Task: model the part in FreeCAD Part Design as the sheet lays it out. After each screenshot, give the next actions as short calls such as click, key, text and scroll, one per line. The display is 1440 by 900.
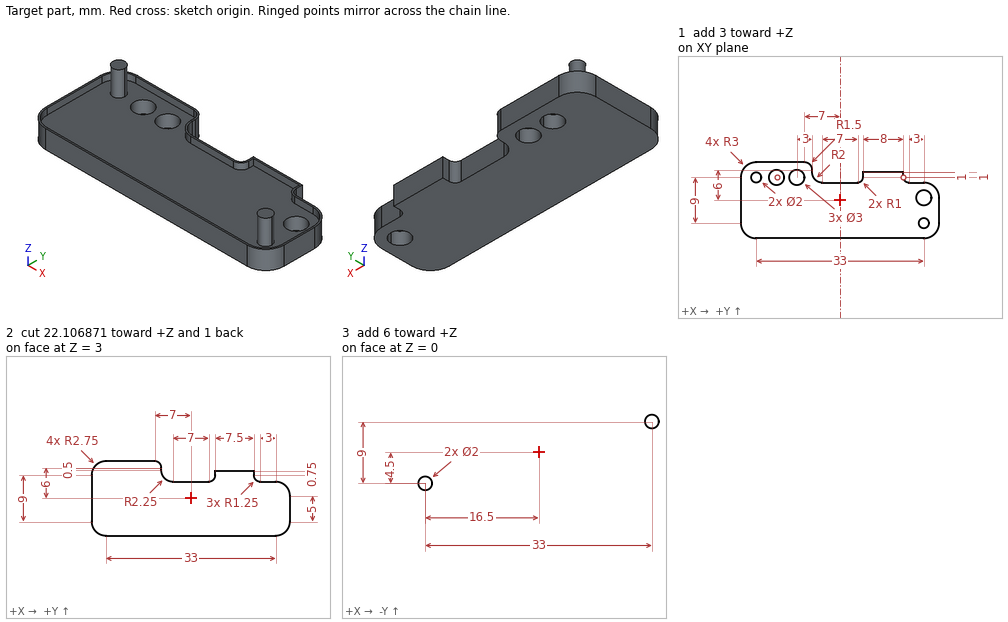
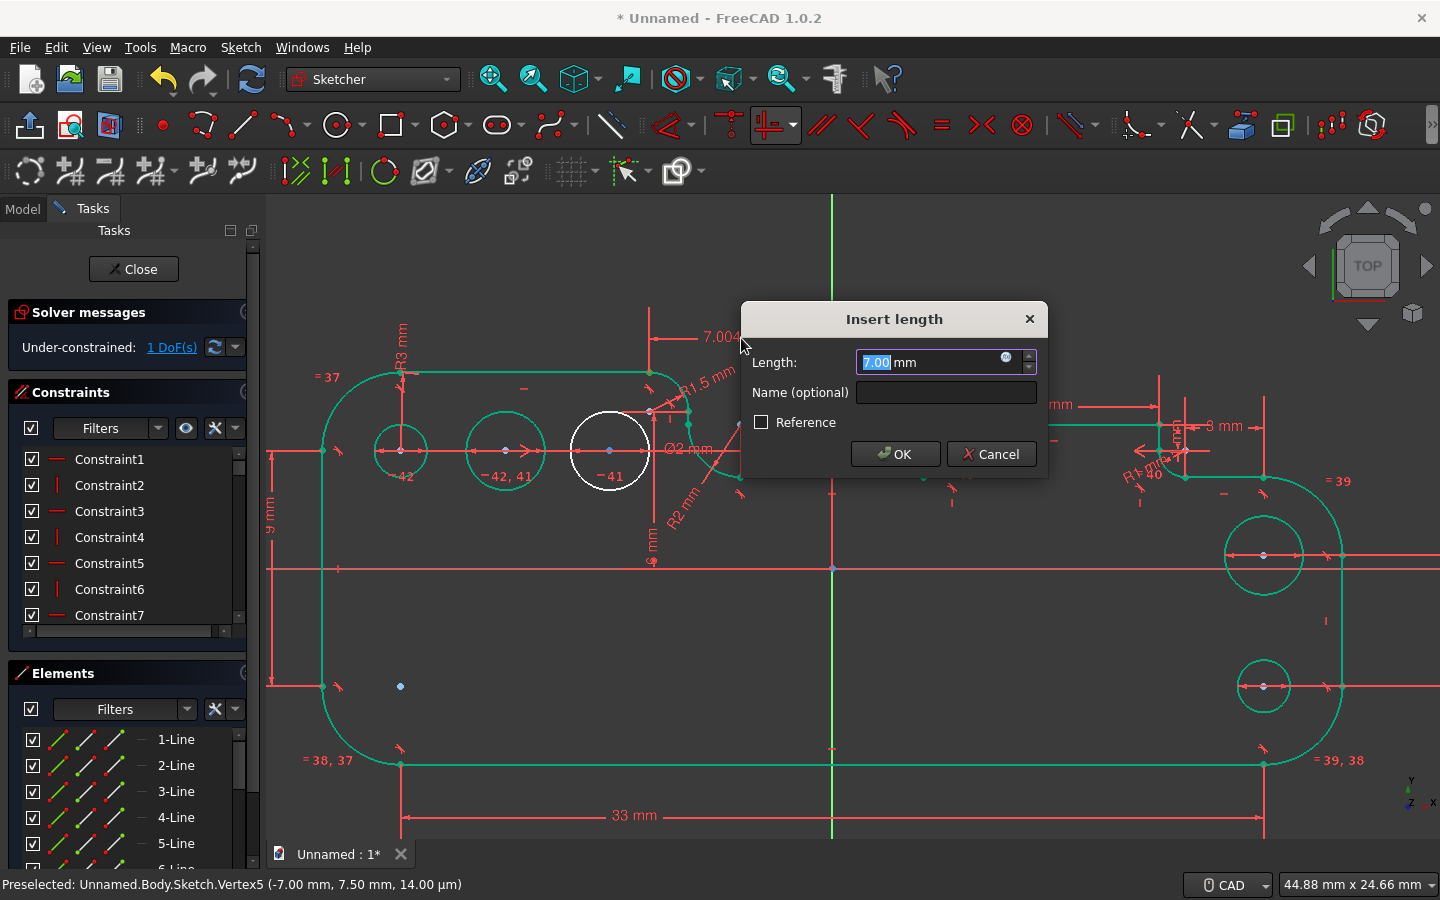
text(7)
key(Return)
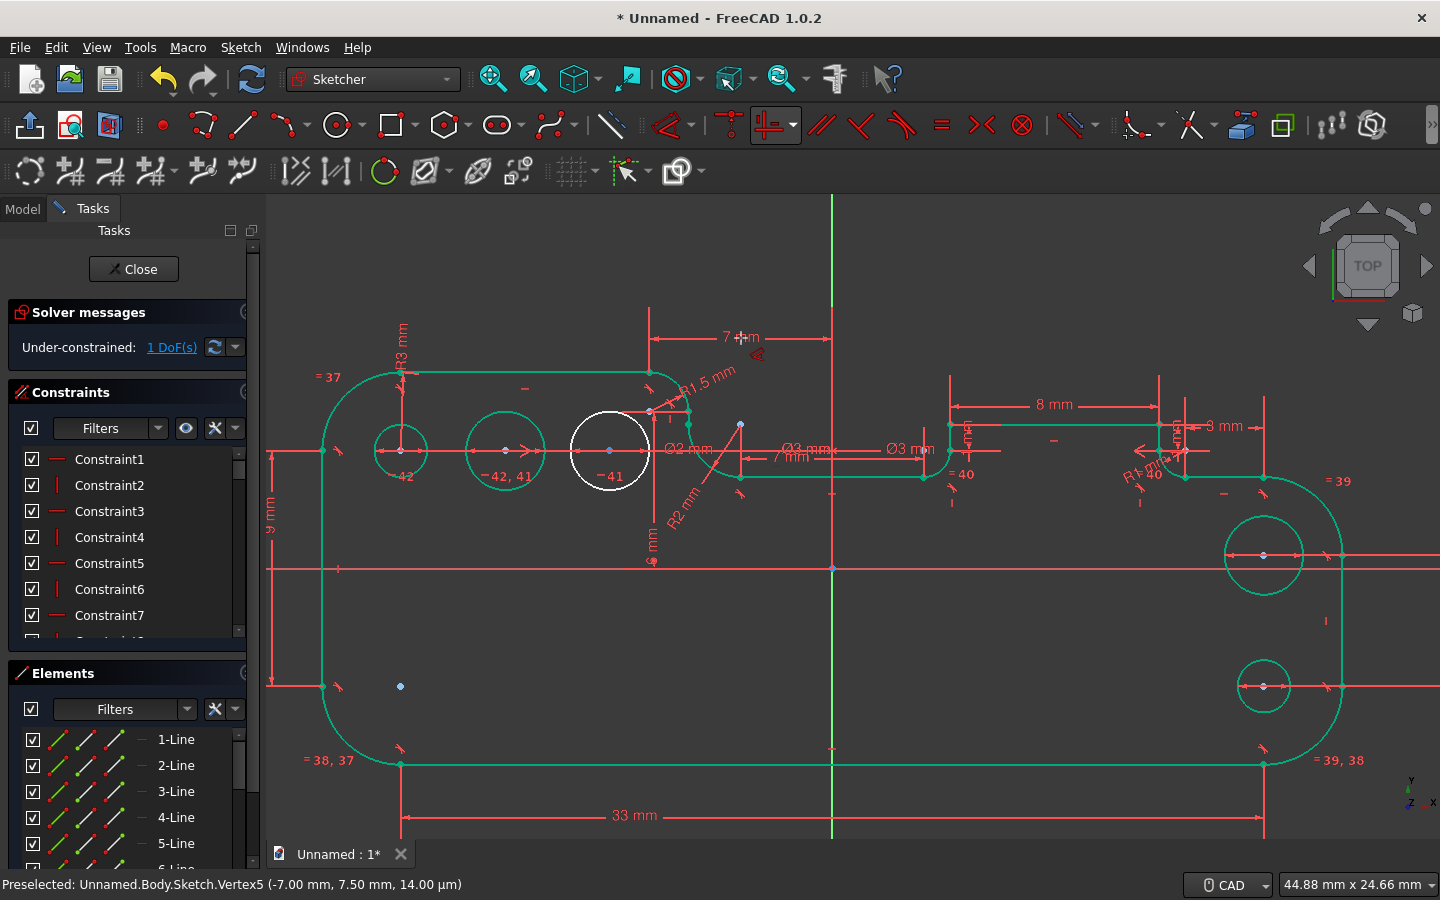
click(689, 425)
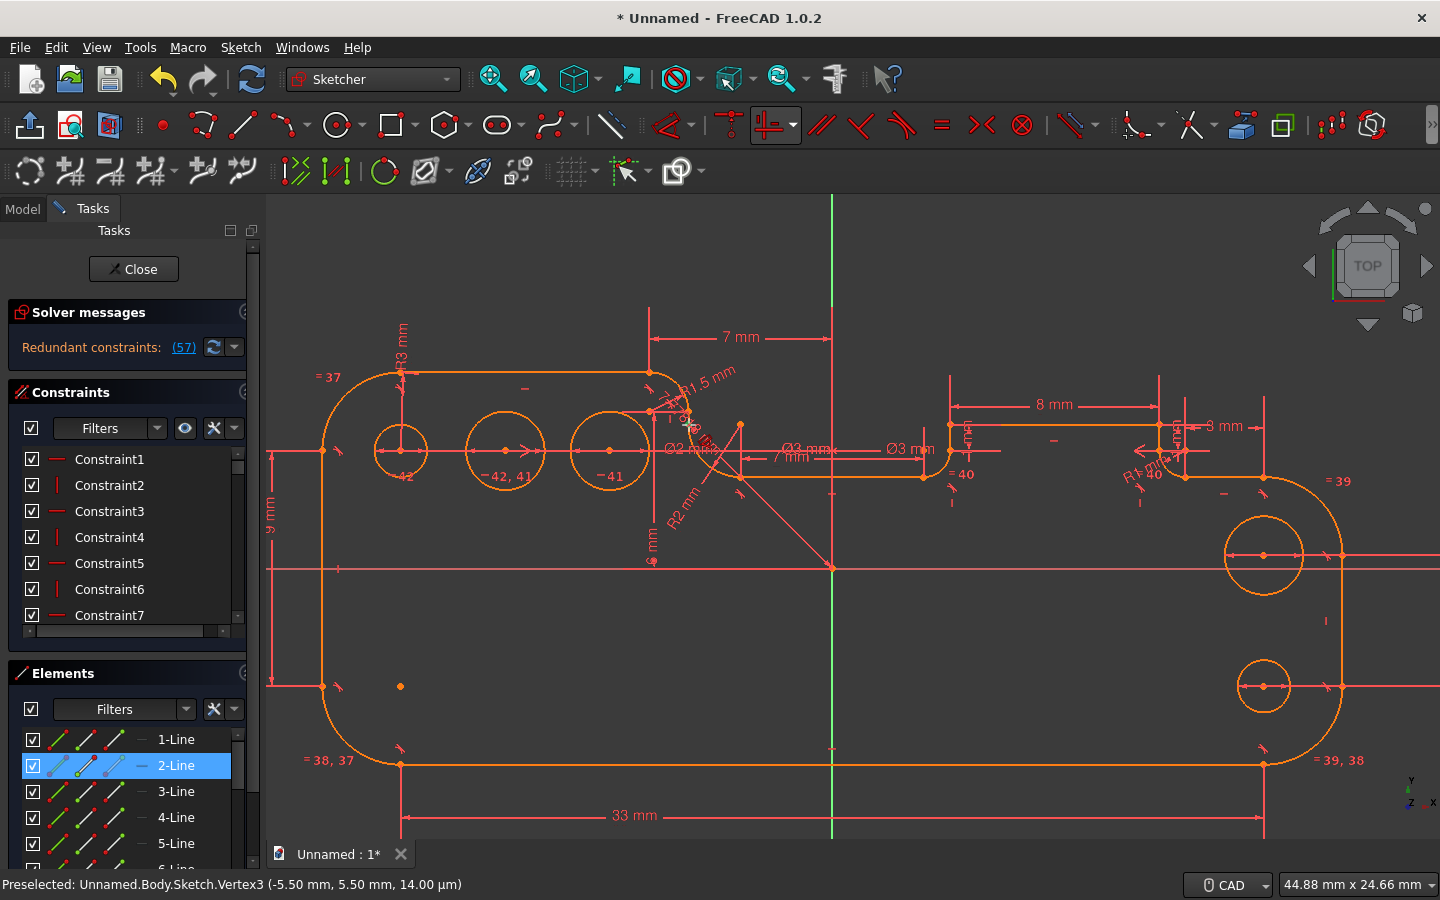
click(610, 451)
click(631, 391)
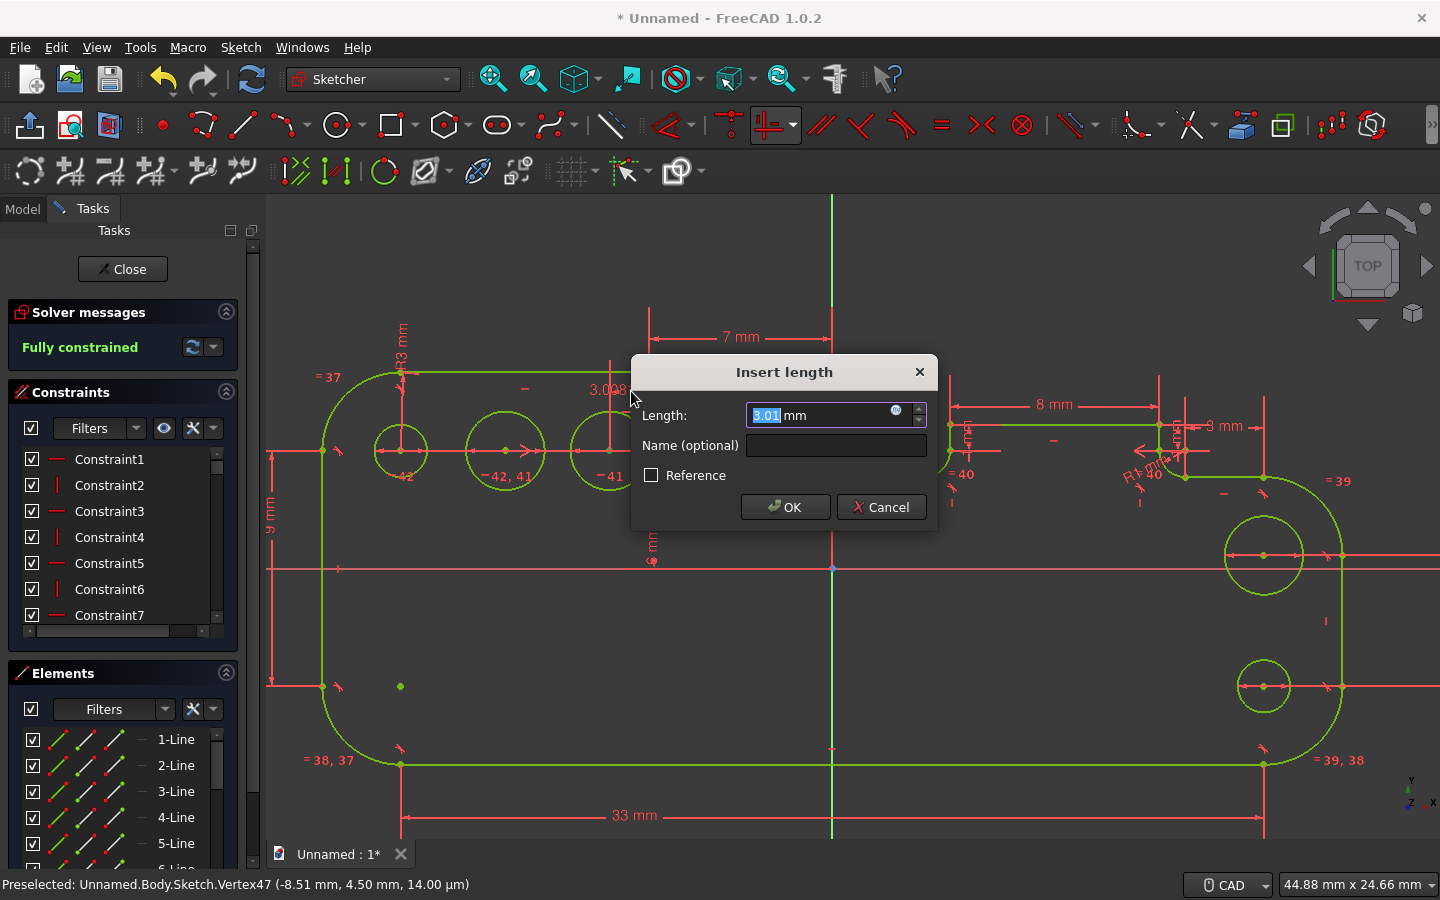
text(3)
key(Return)
key(Escape)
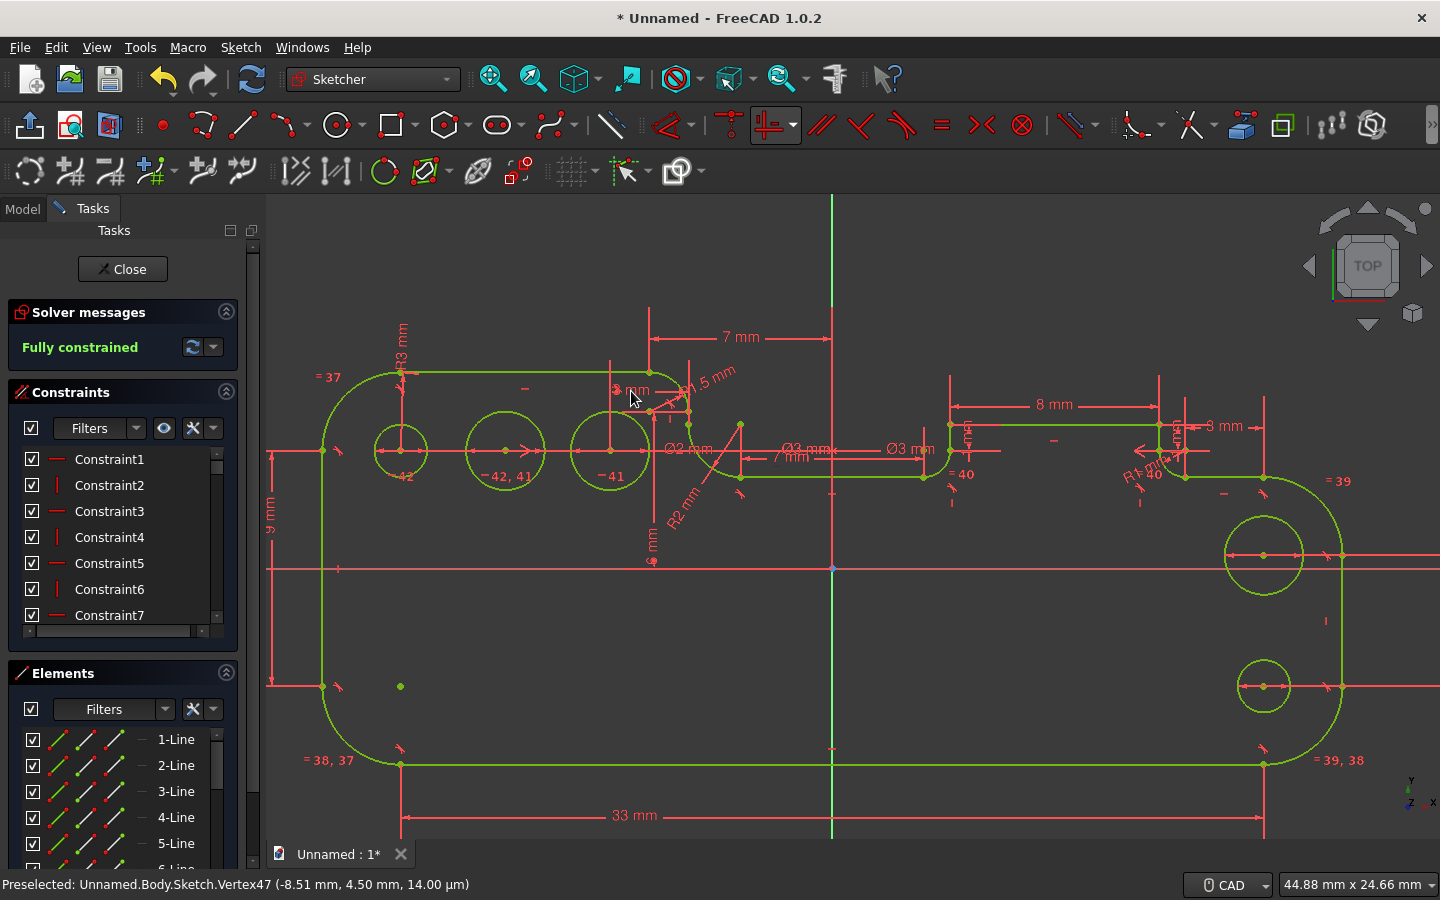
click(123, 269)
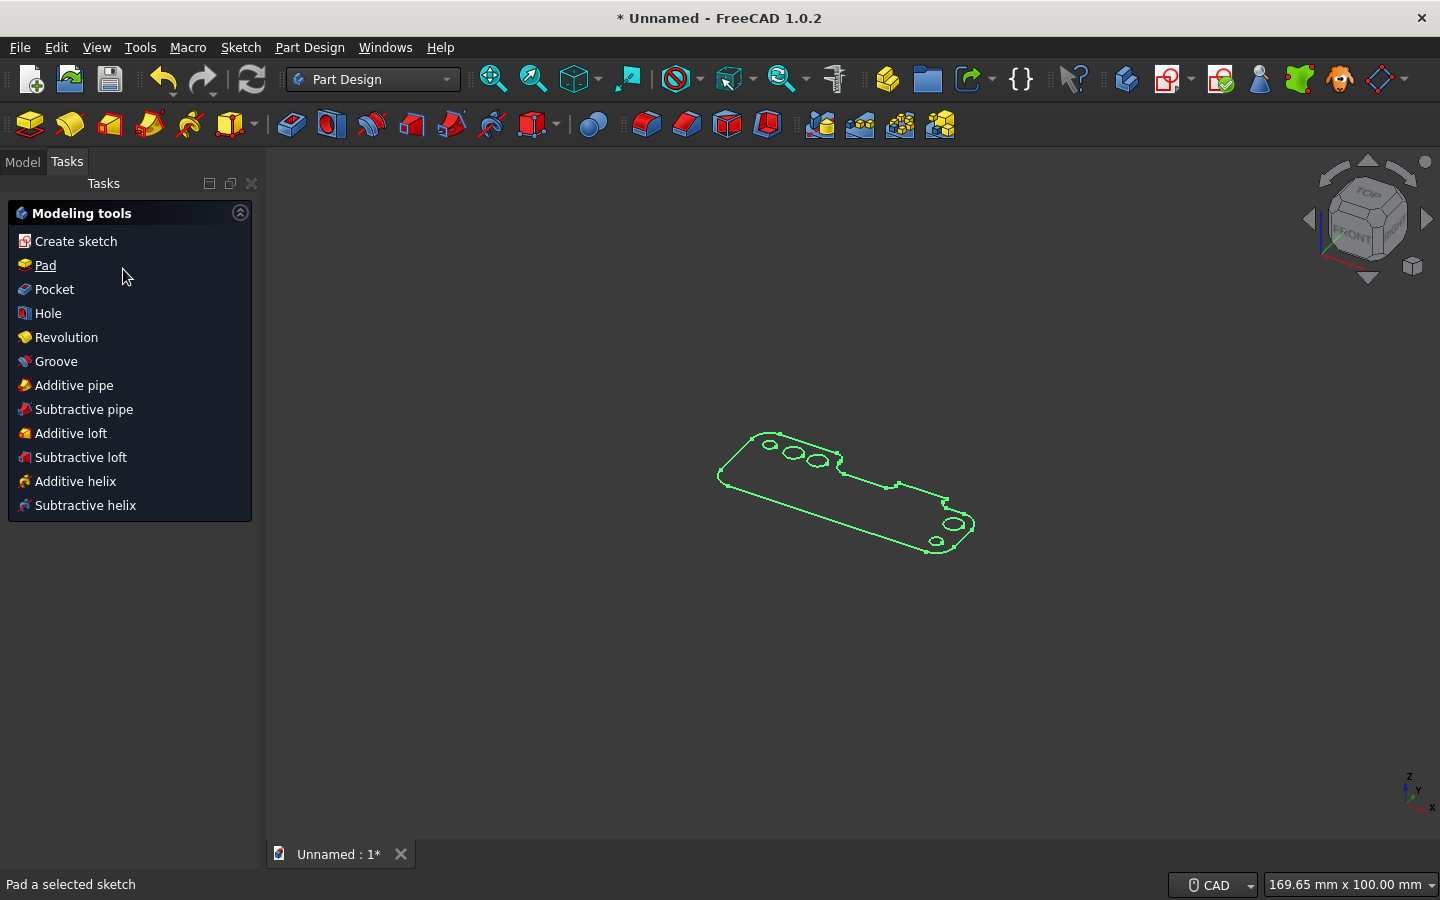
click(30, 124)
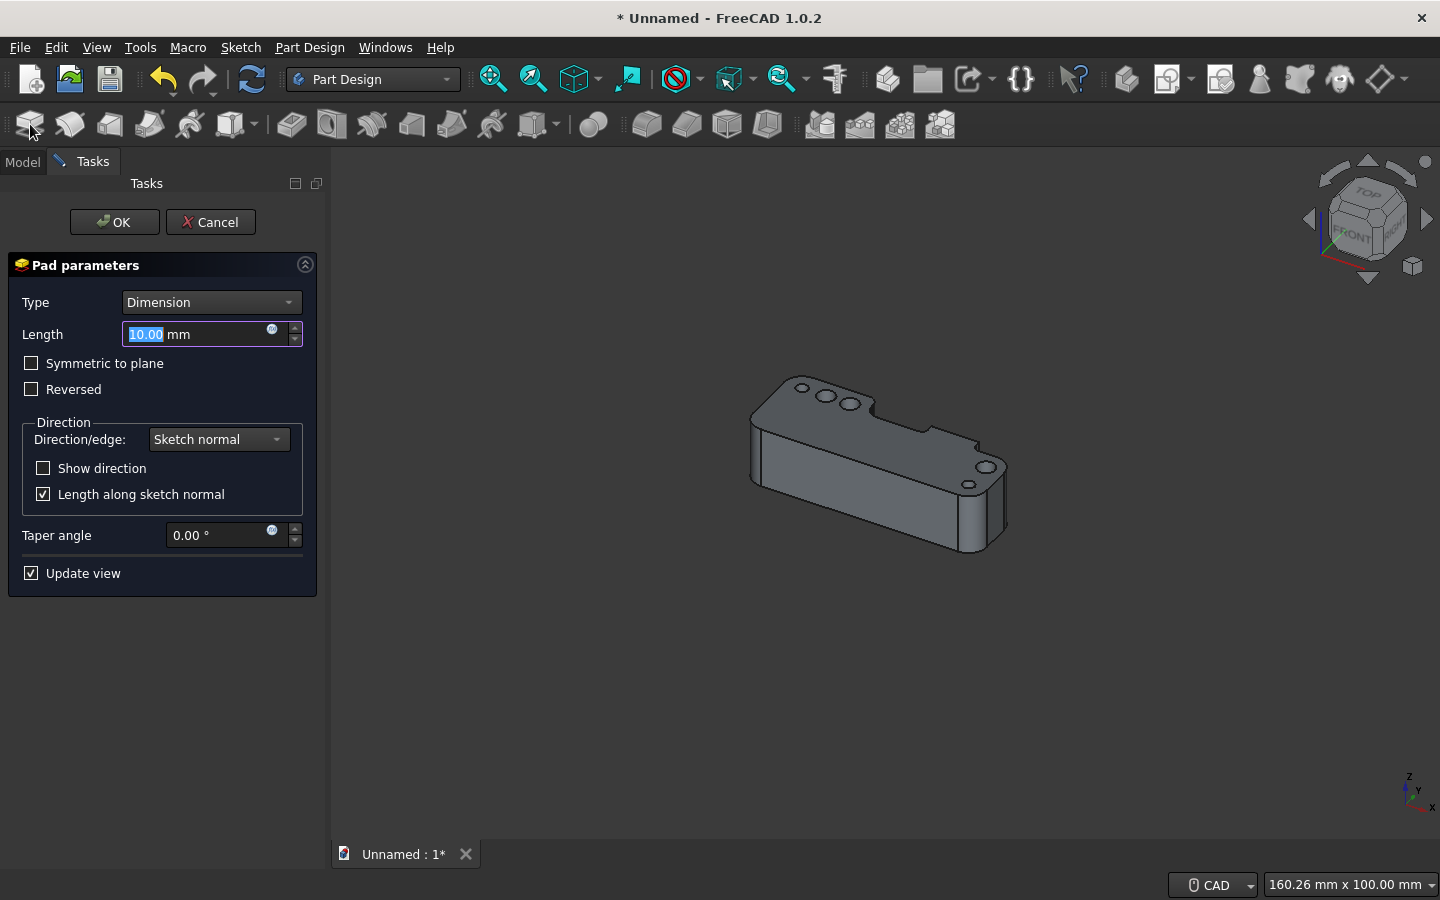
text(3)
key(Tab)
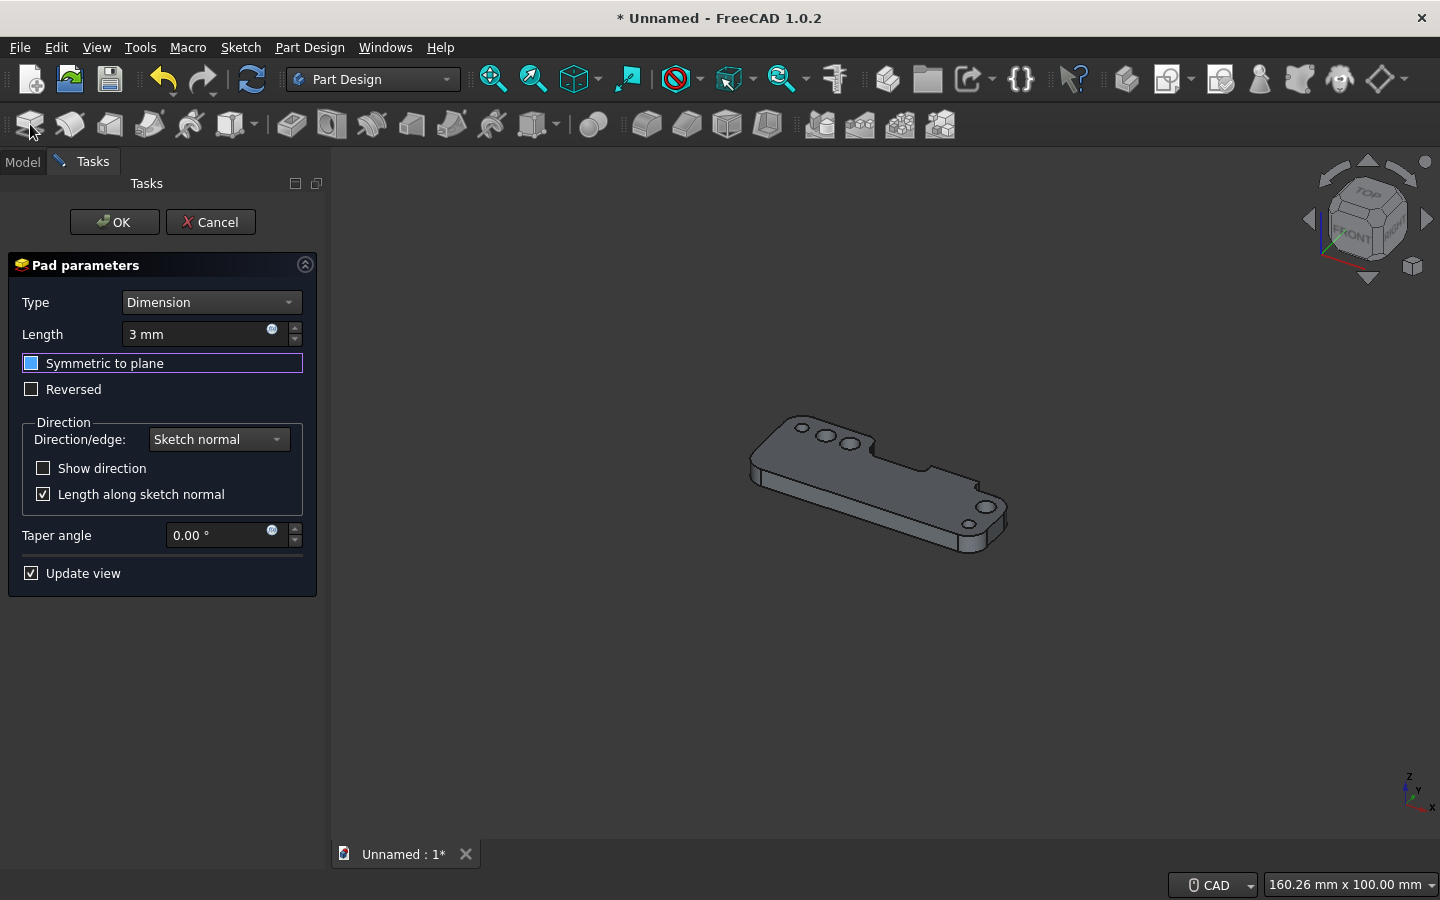
click(115, 222)